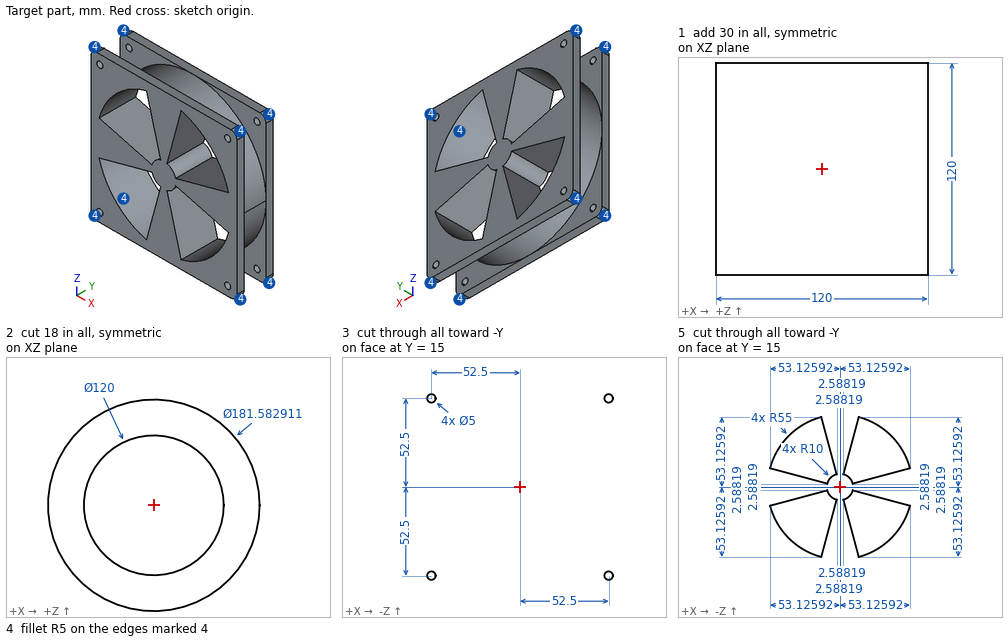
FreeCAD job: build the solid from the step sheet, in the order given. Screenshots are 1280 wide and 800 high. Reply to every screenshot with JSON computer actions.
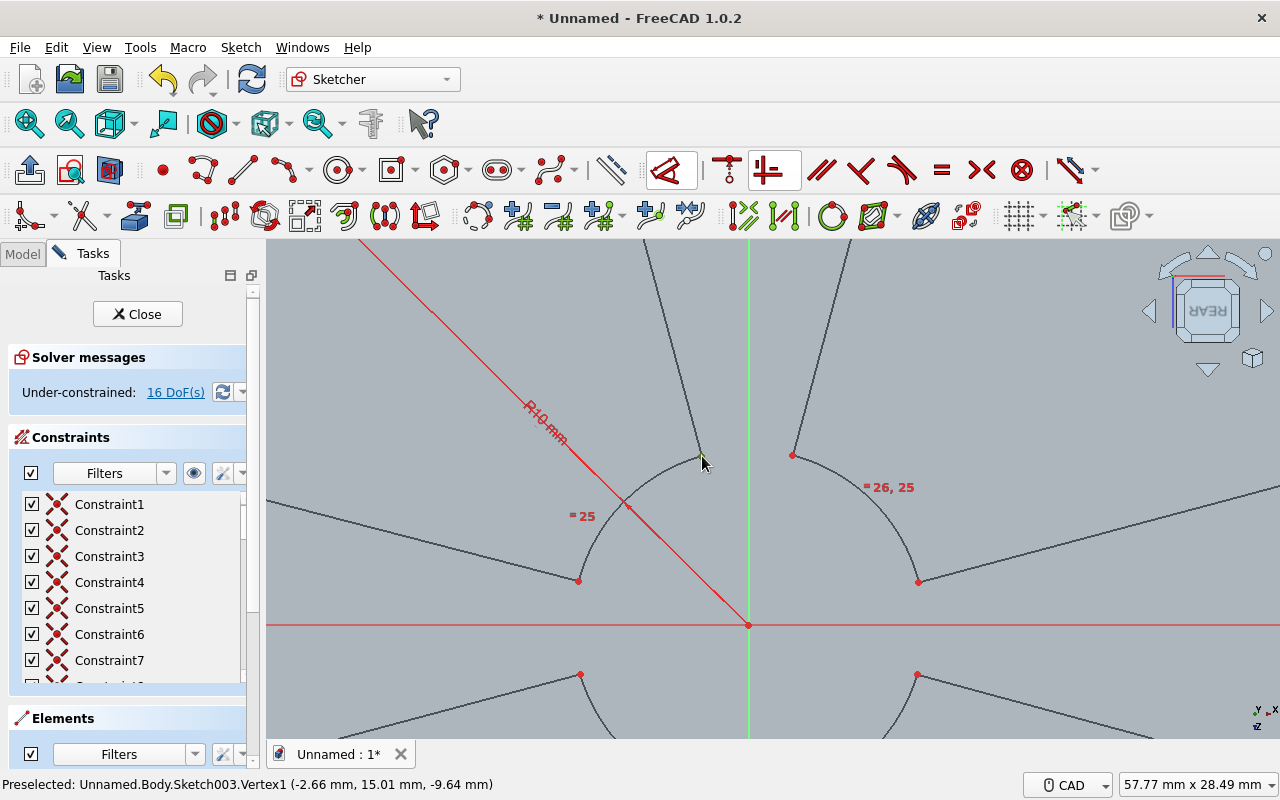
{"action": "left_click", "coordinate": [692, 170]}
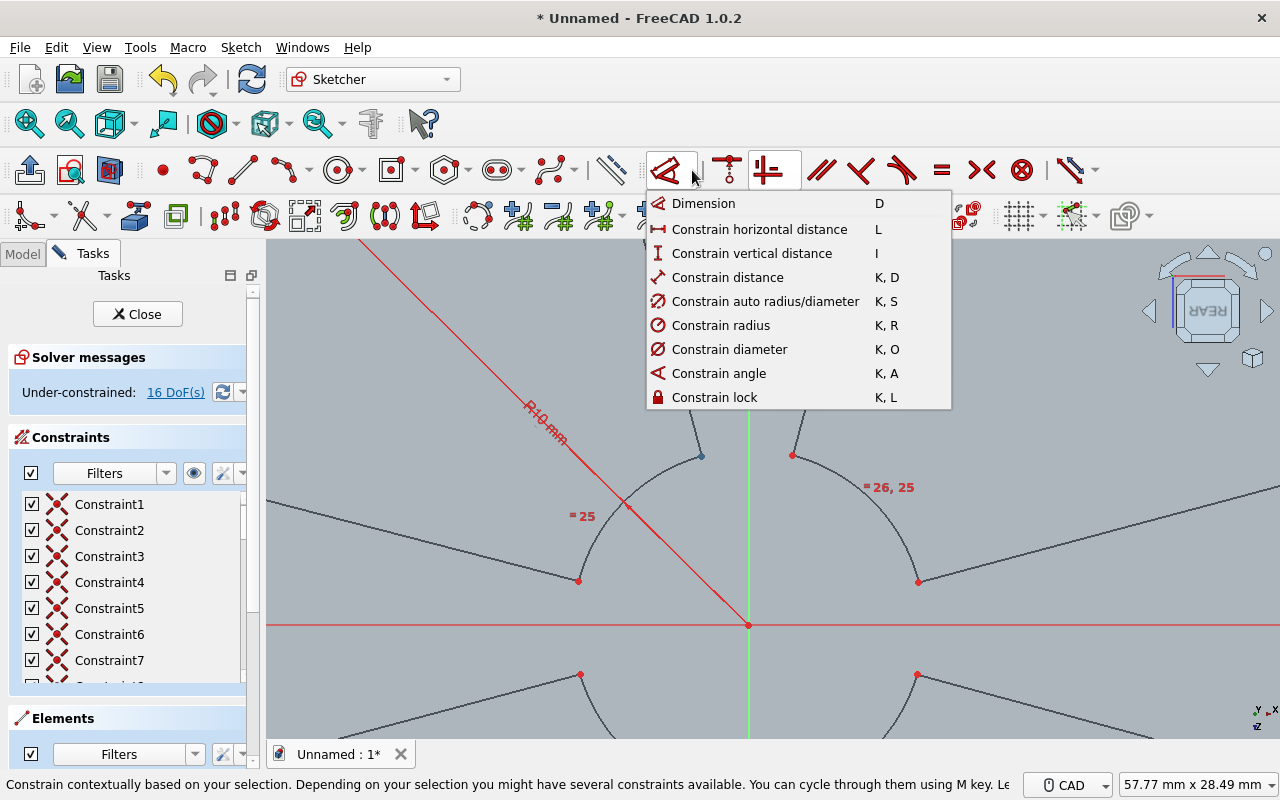
{"action": "left_click", "coordinate": [799, 229]}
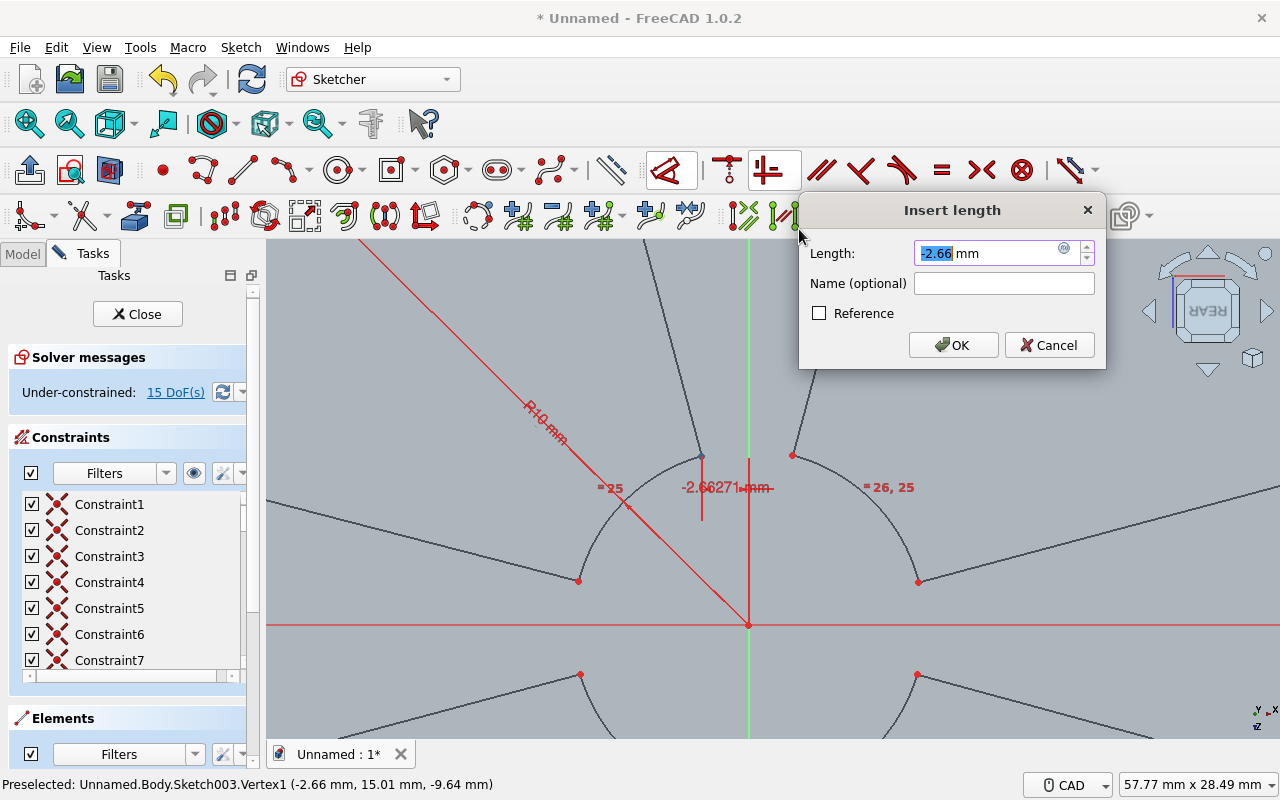
{"action": "type", "text": "-2.58819"}
{"action": "key", "text": "Return"}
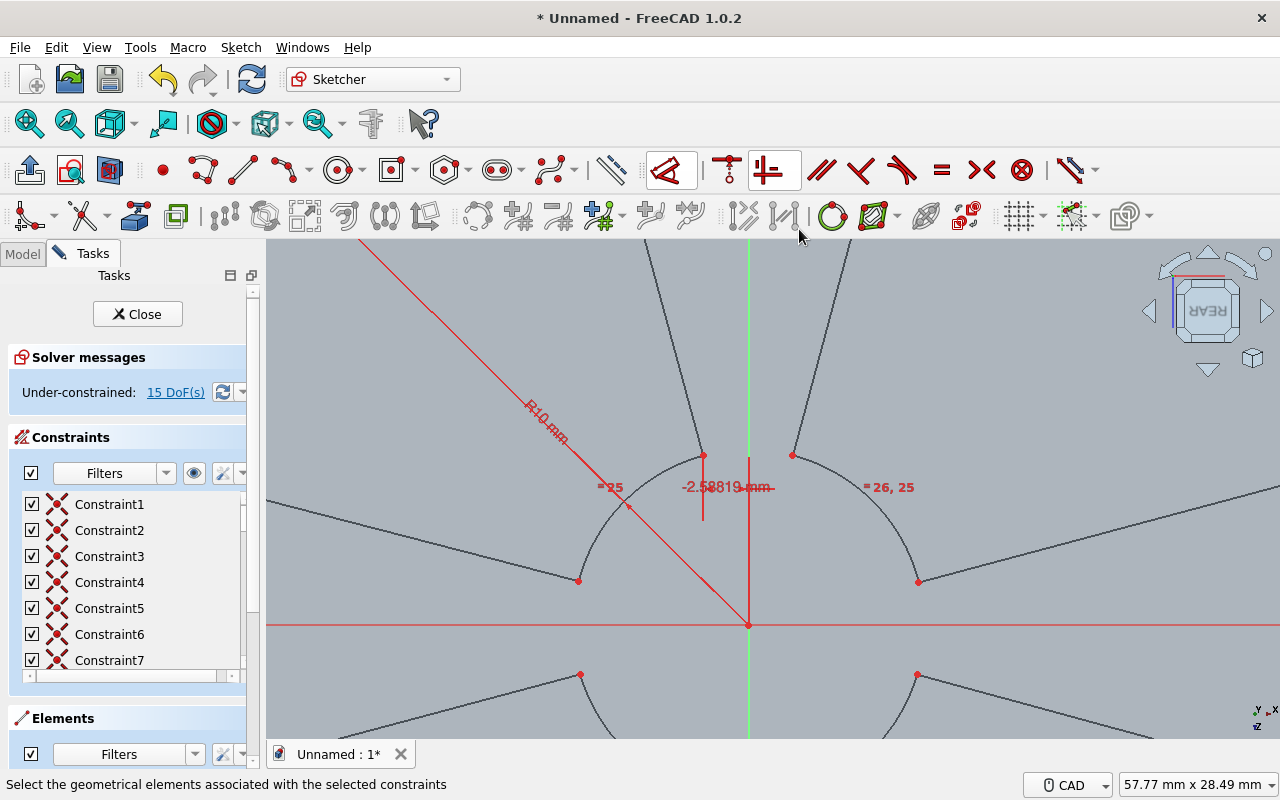
{"action": "left_click", "coordinate": [579, 581]}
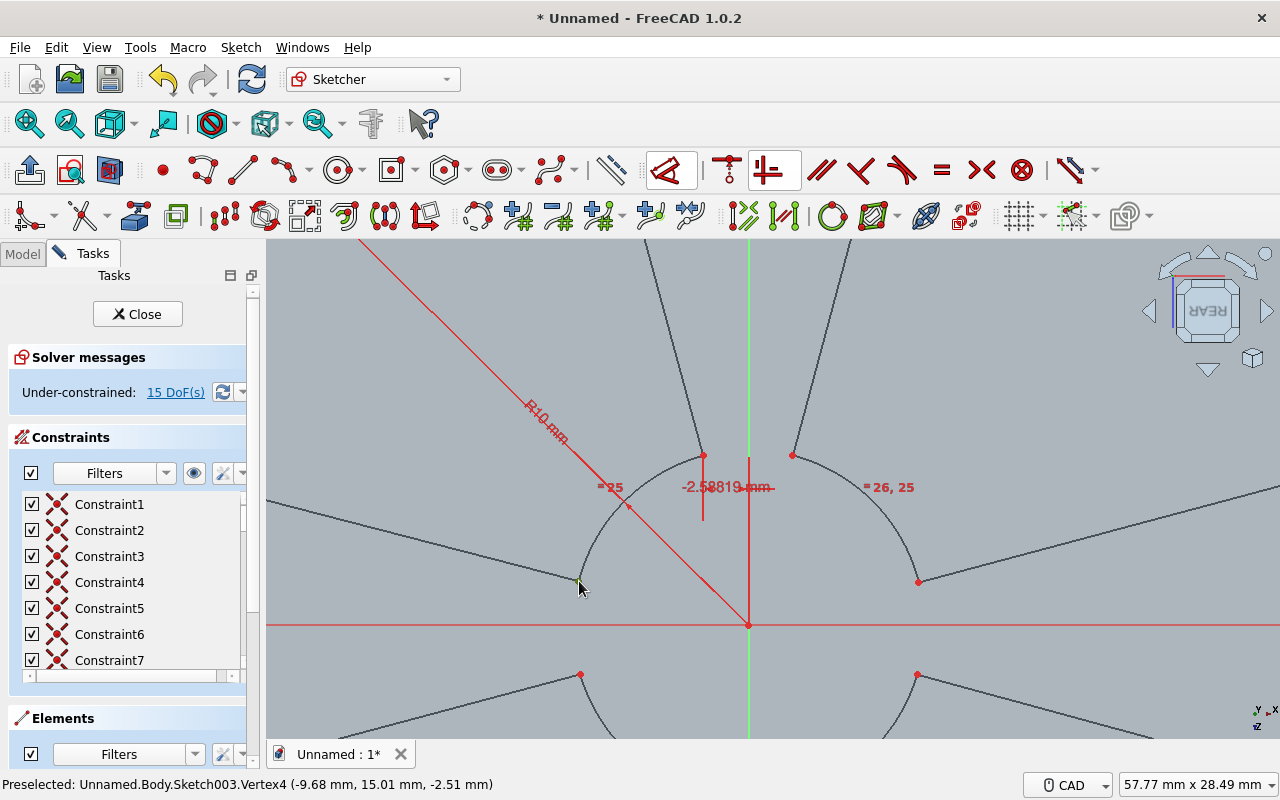
{"action": "left_click", "coordinate": [692, 170]}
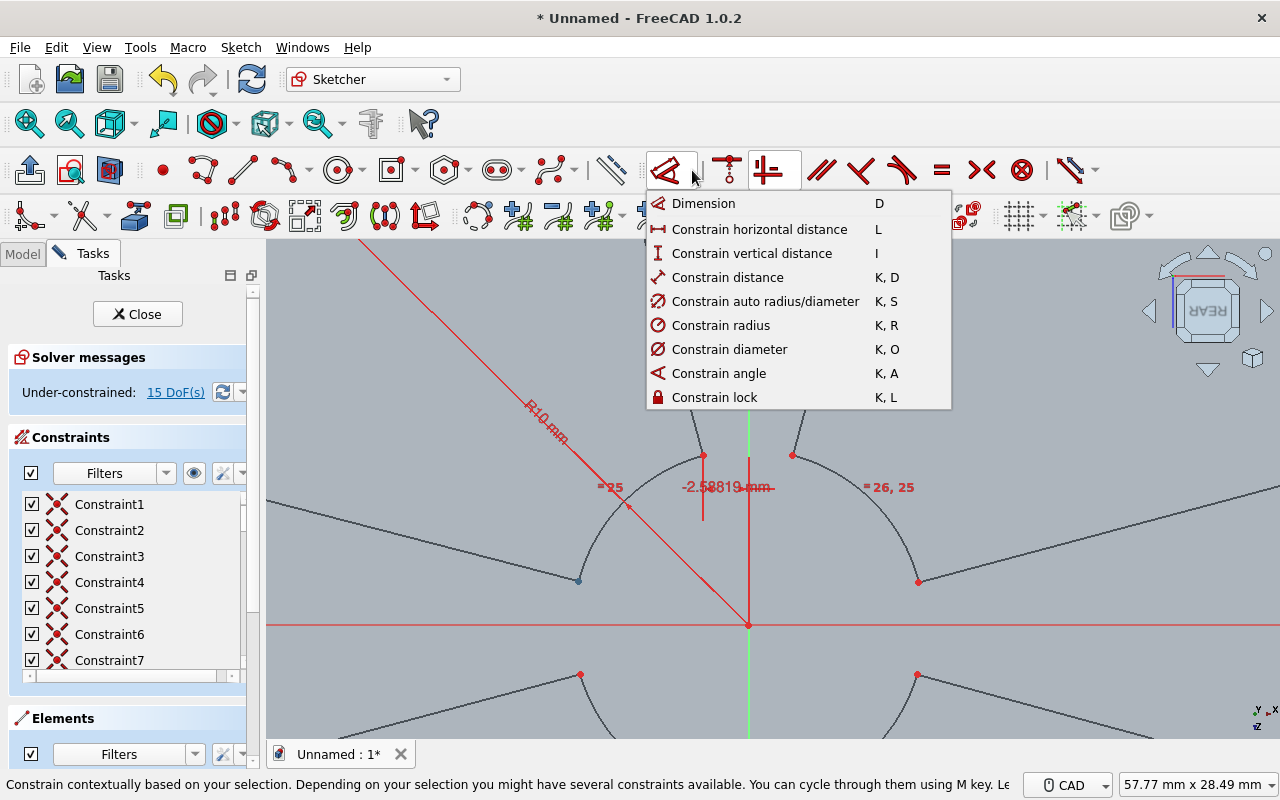
{"action": "left_click", "coordinate": [799, 253]}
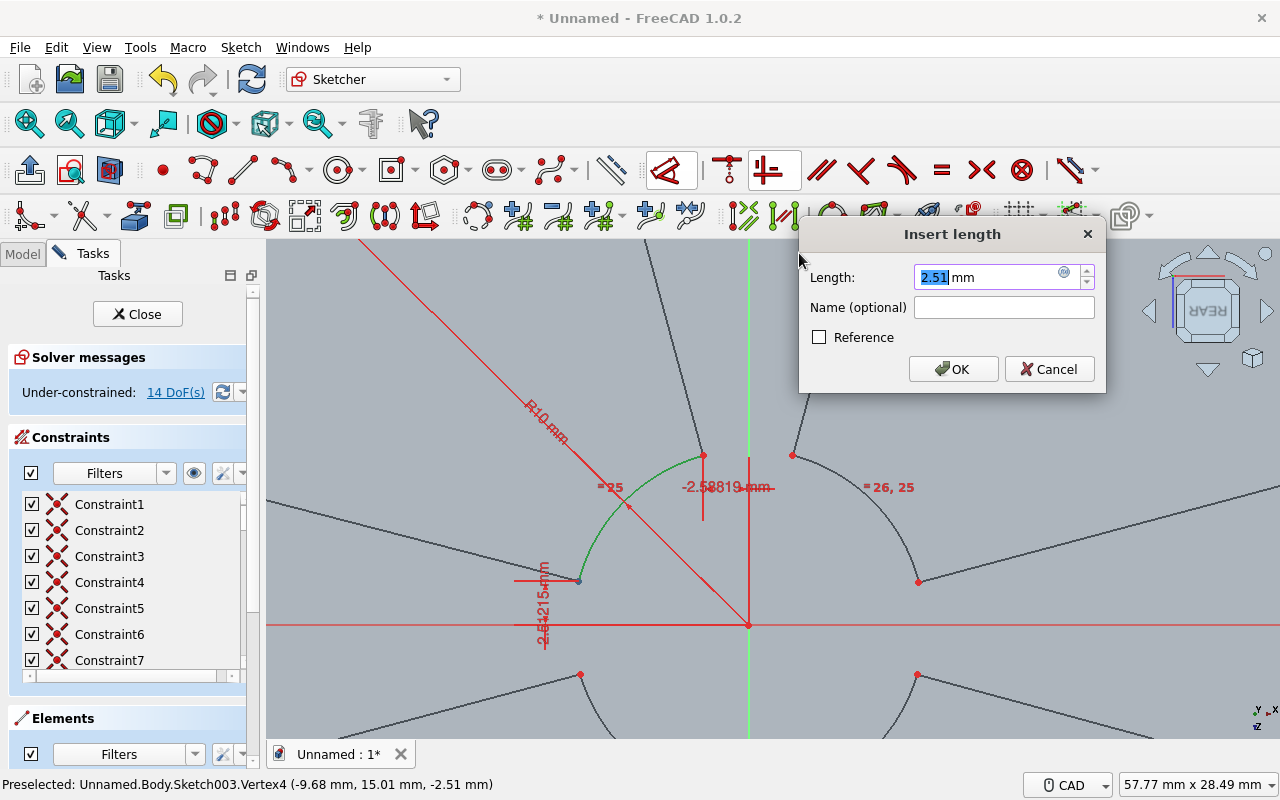
{"action": "type", "text": "2.58819"}
{"action": "key", "text": "Return"}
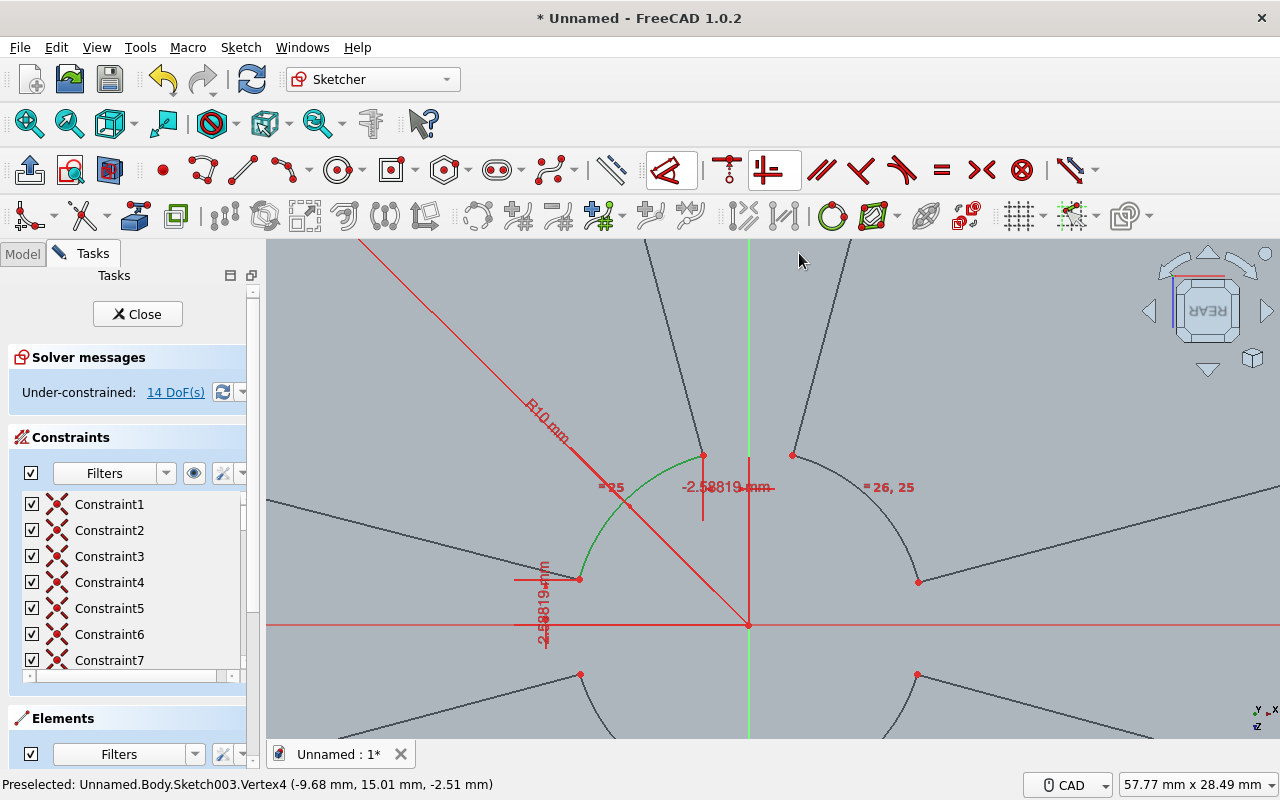
{"action": "left_click", "coordinate": [793, 455]}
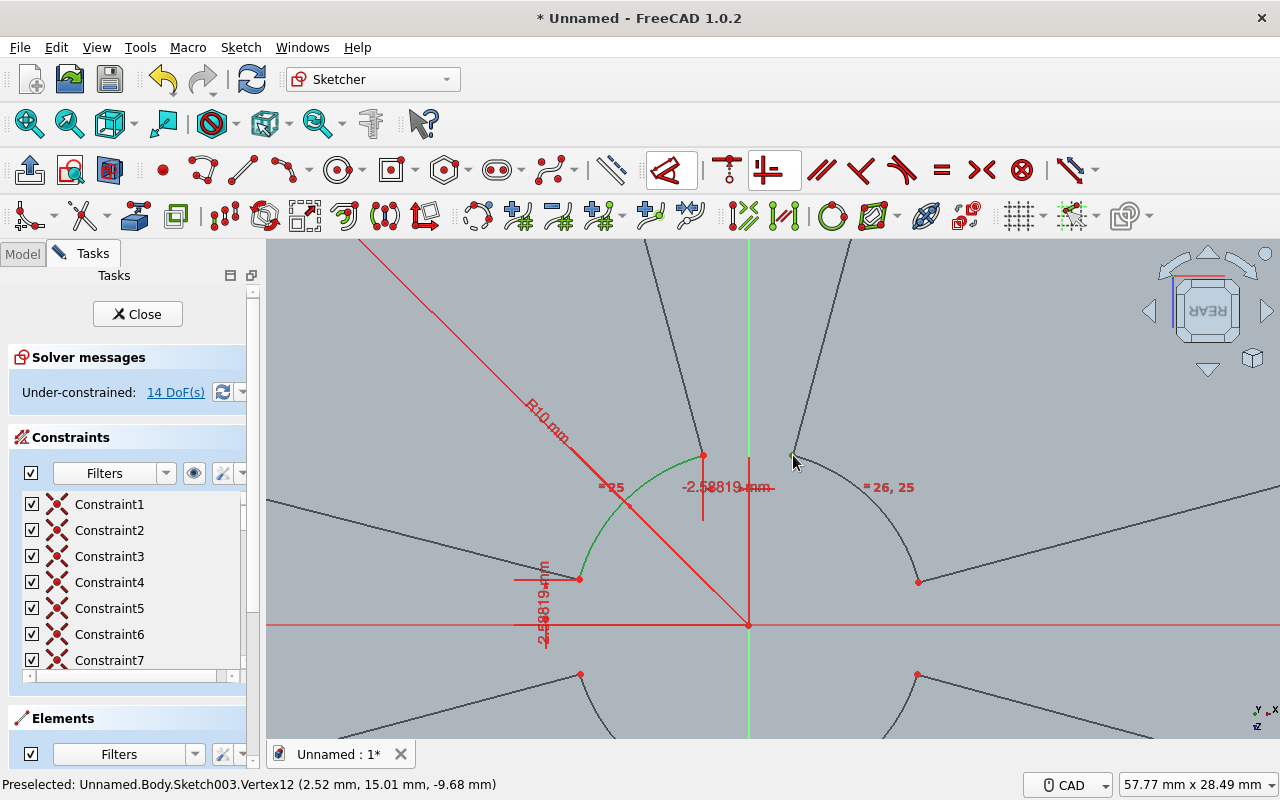
{"action": "key", "text": "l"}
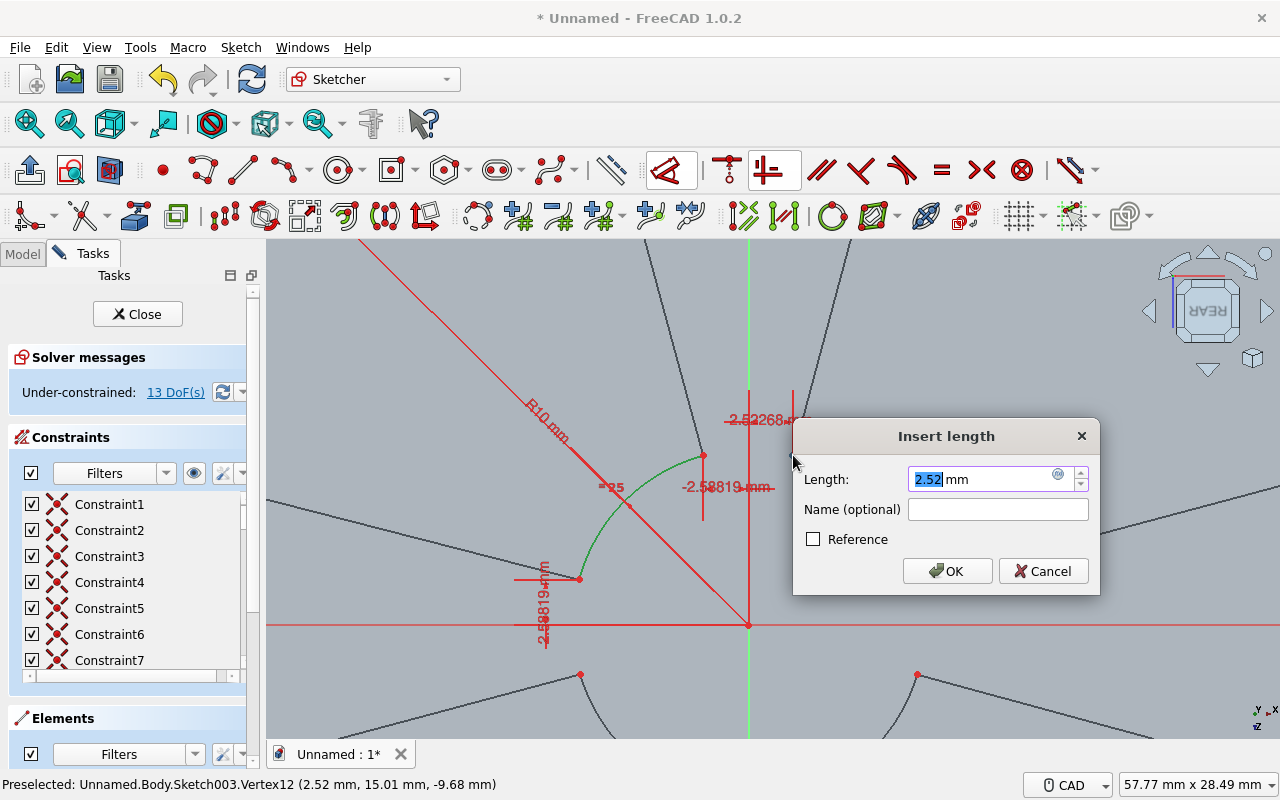
{"action": "type", "text": "2.58819"}
{"action": "key", "text": "Return"}